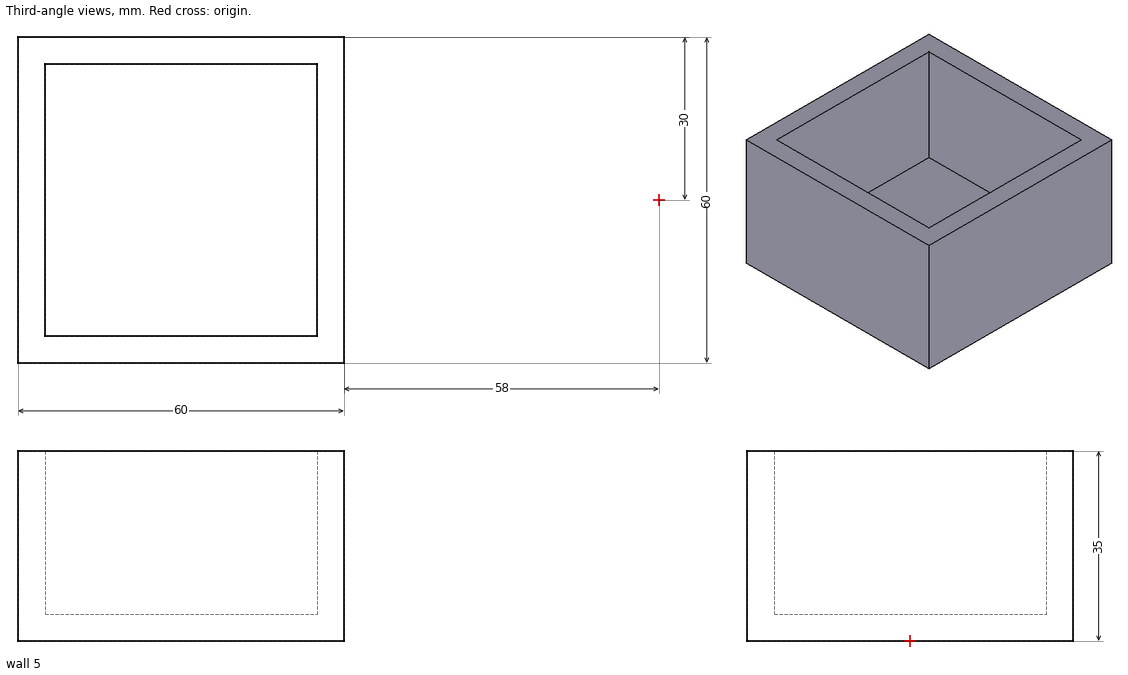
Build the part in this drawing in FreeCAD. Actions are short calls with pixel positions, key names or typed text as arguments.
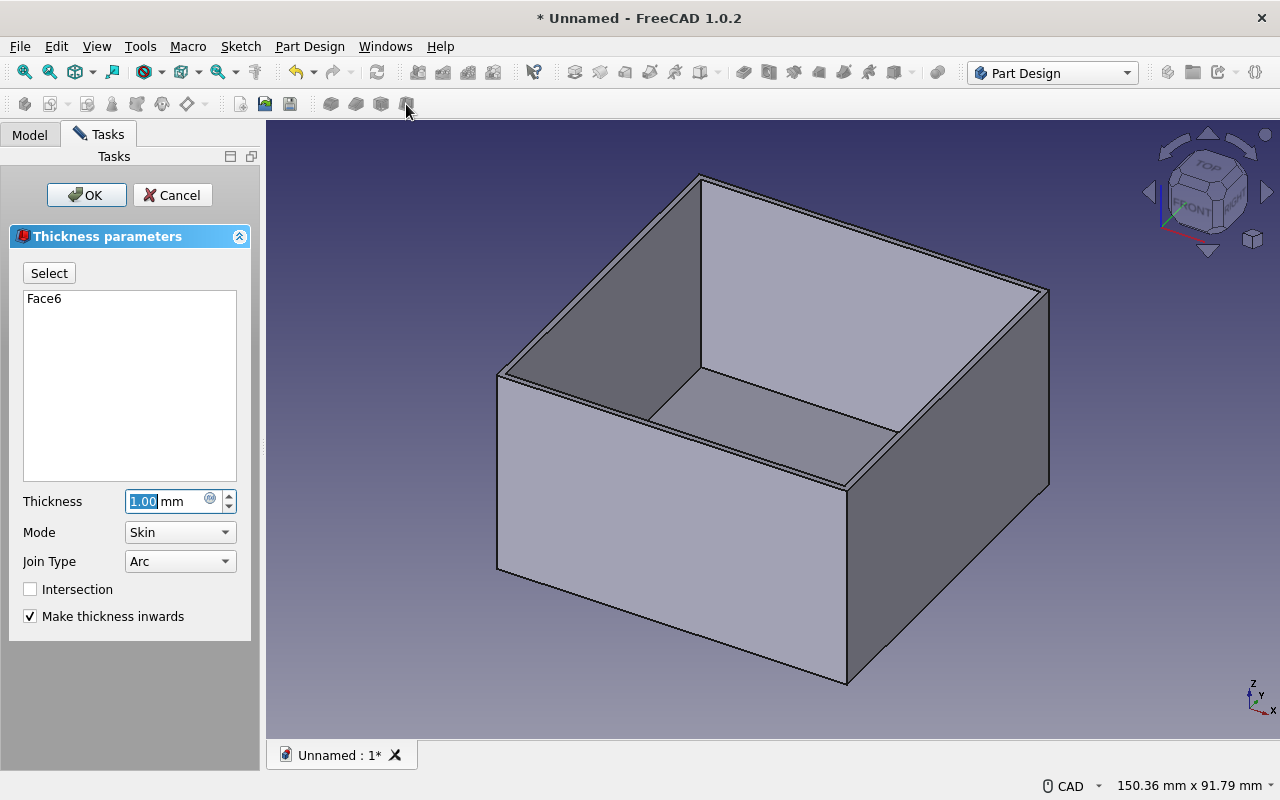
text(5)
key(Tab)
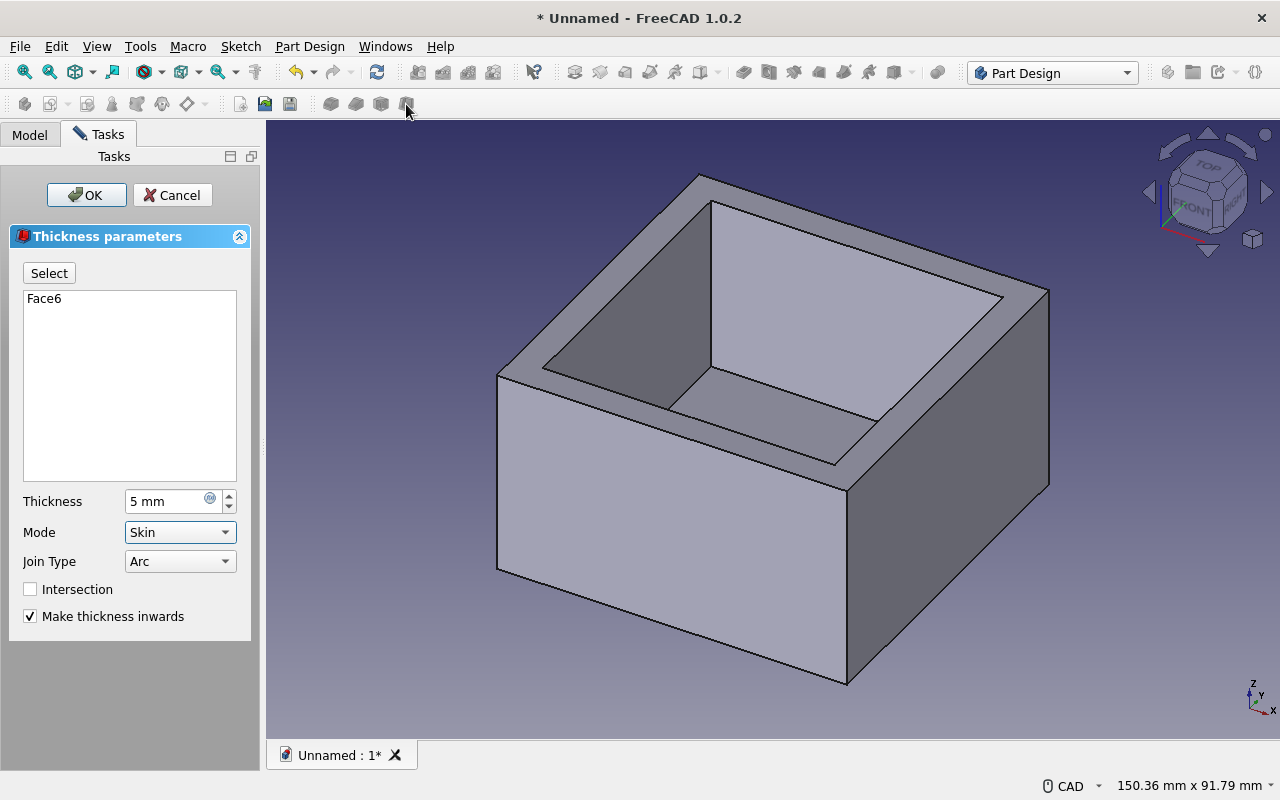
click(181, 562)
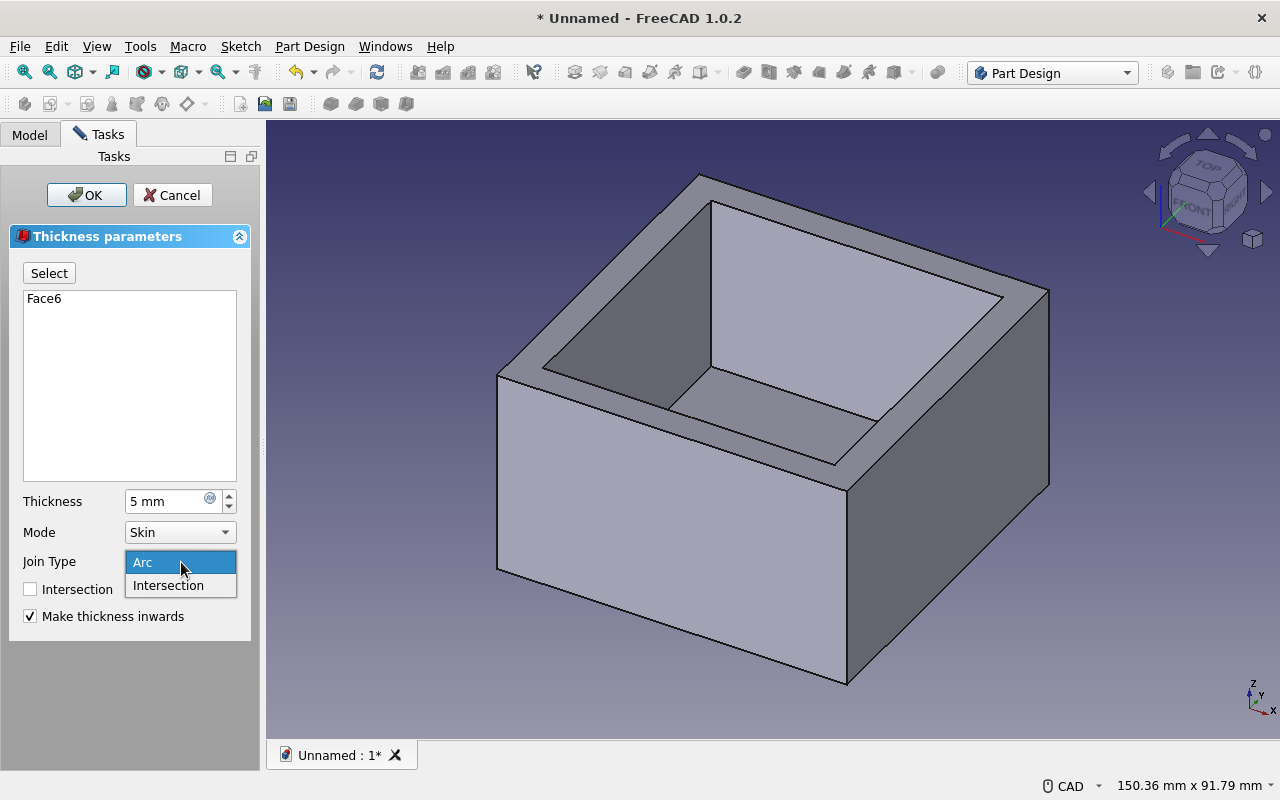
click(179, 586)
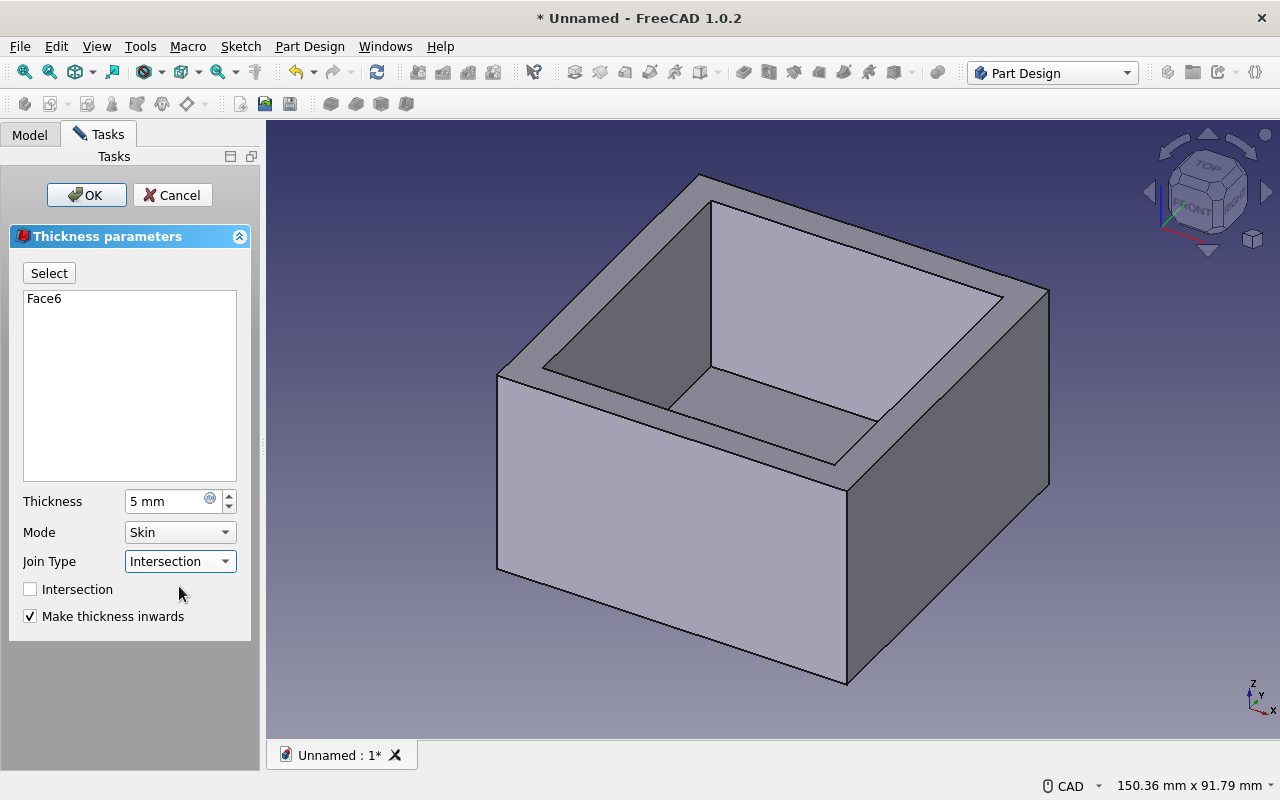
click(87, 195)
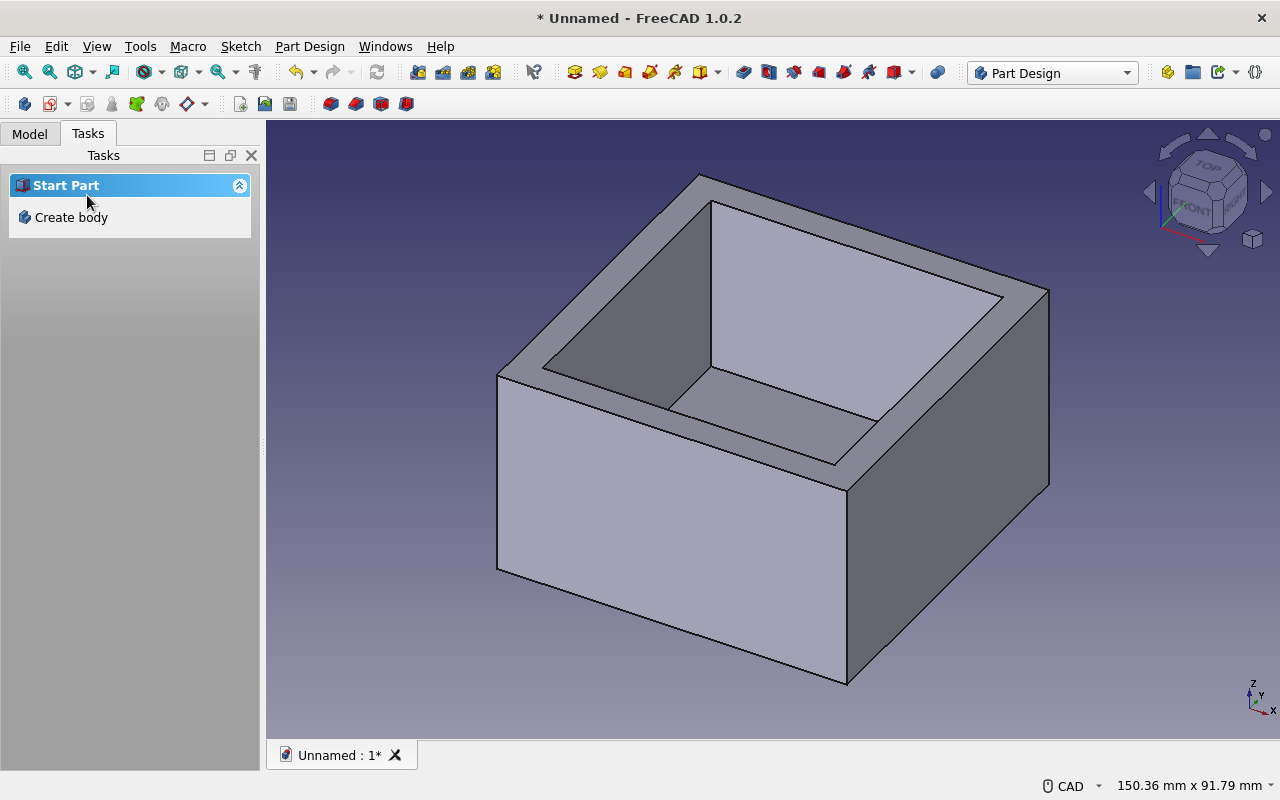
key(0)